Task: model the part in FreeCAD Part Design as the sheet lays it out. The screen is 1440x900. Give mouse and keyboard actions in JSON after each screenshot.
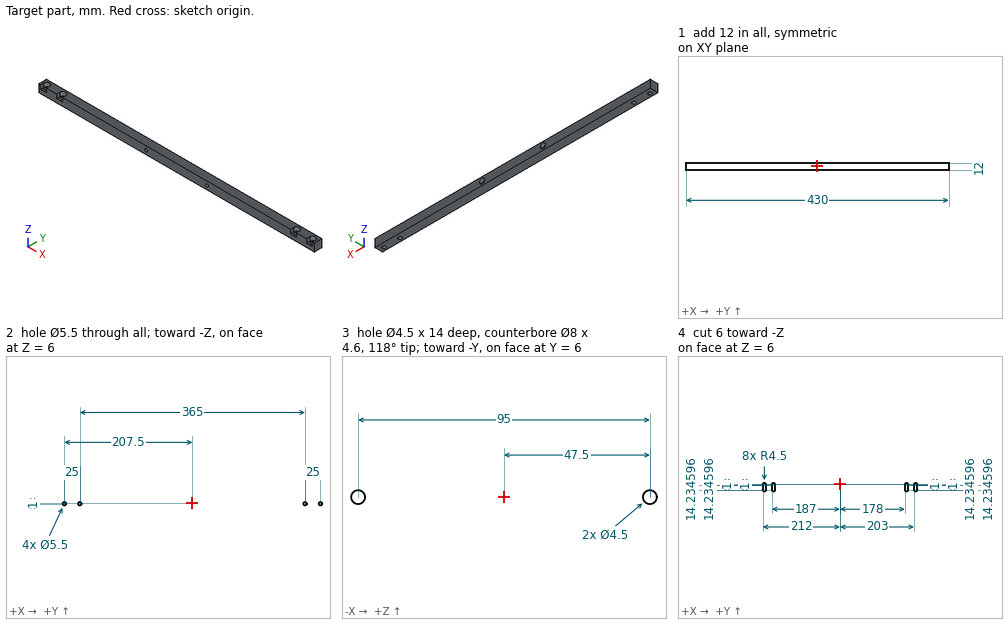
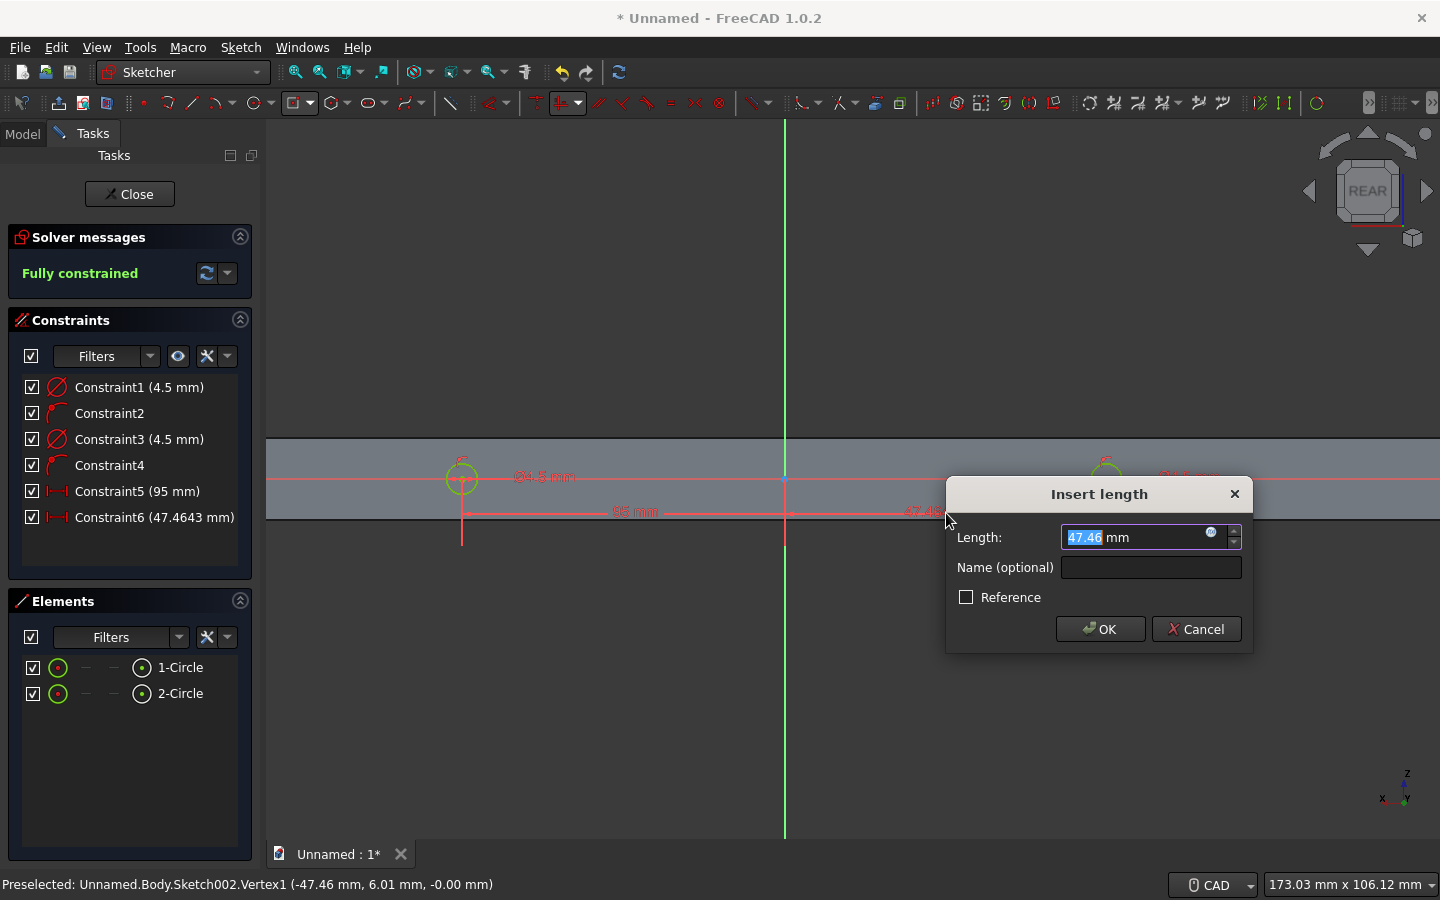
{"action": "type", "text": "47.5"}
{"action": "key", "text": "Return"}
{"action": "key", "text": "Escape"}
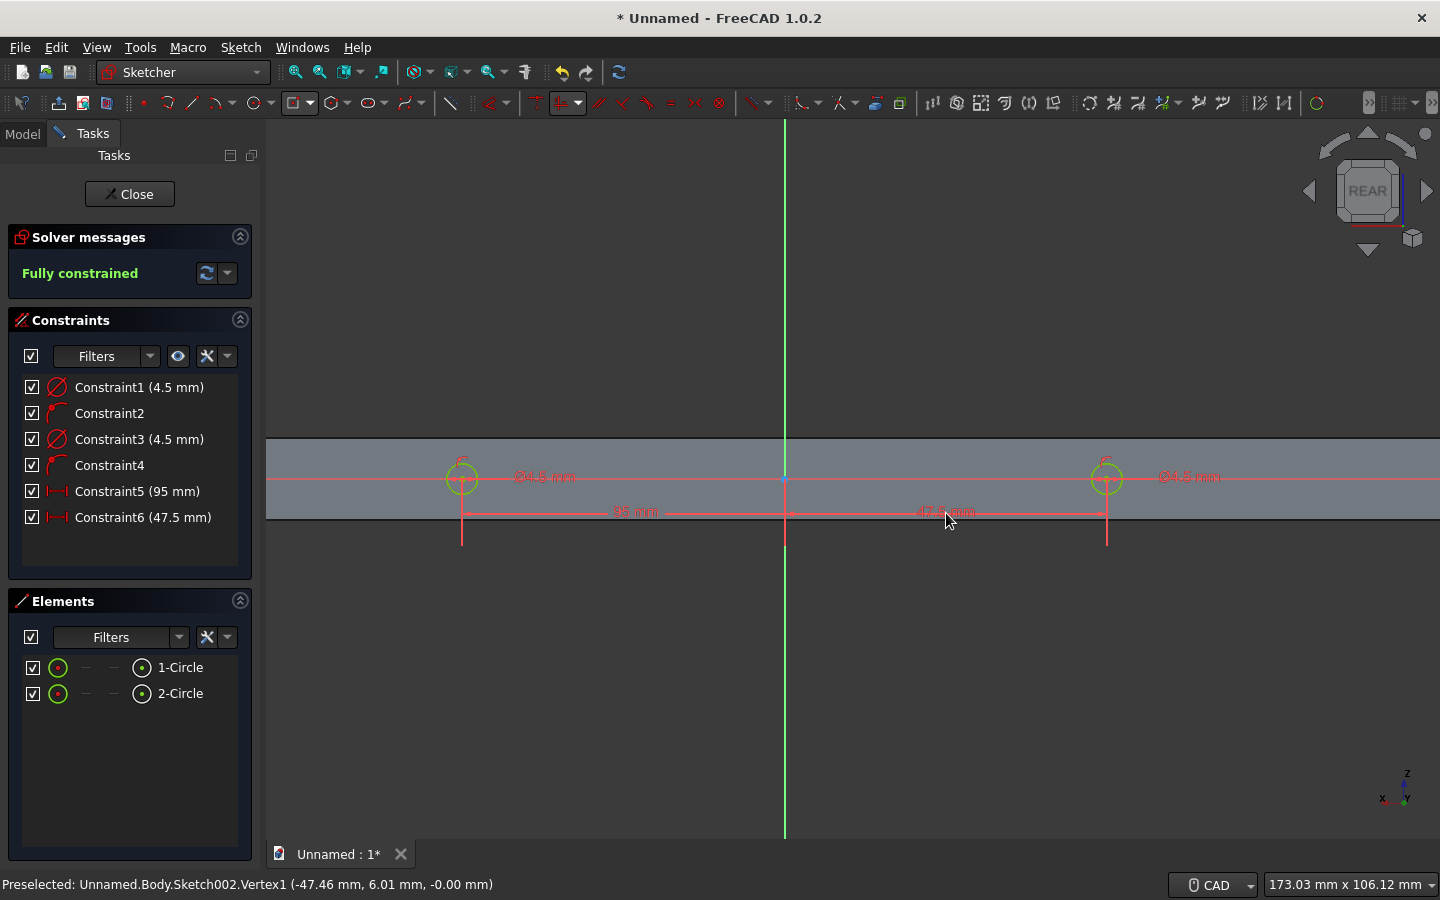
{"action": "left_click", "coordinate": [130, 194]}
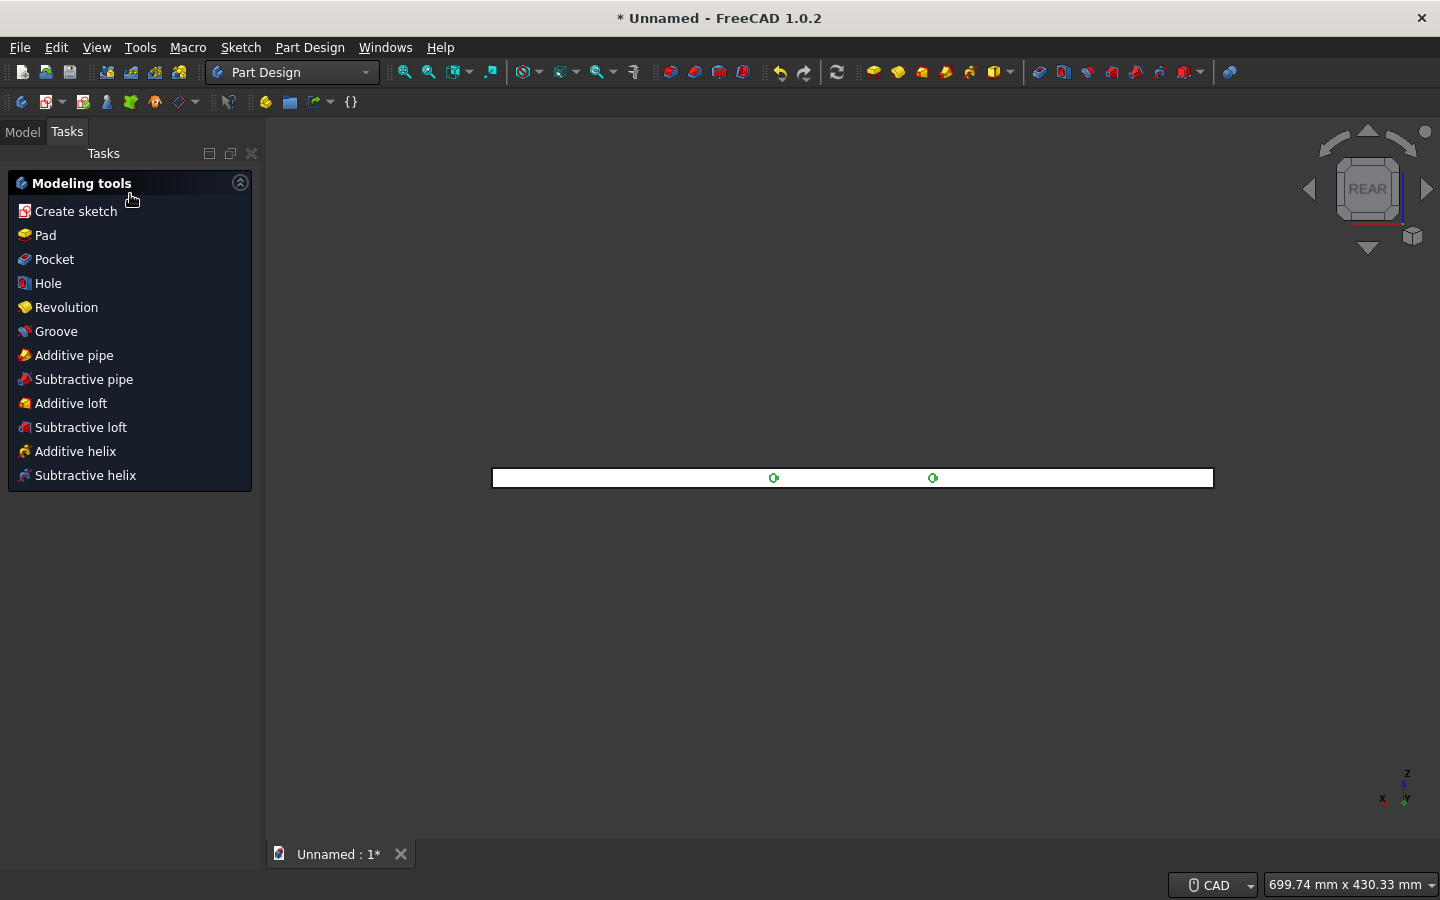
{"action": "left_click", "coordinate": [1064, 72]}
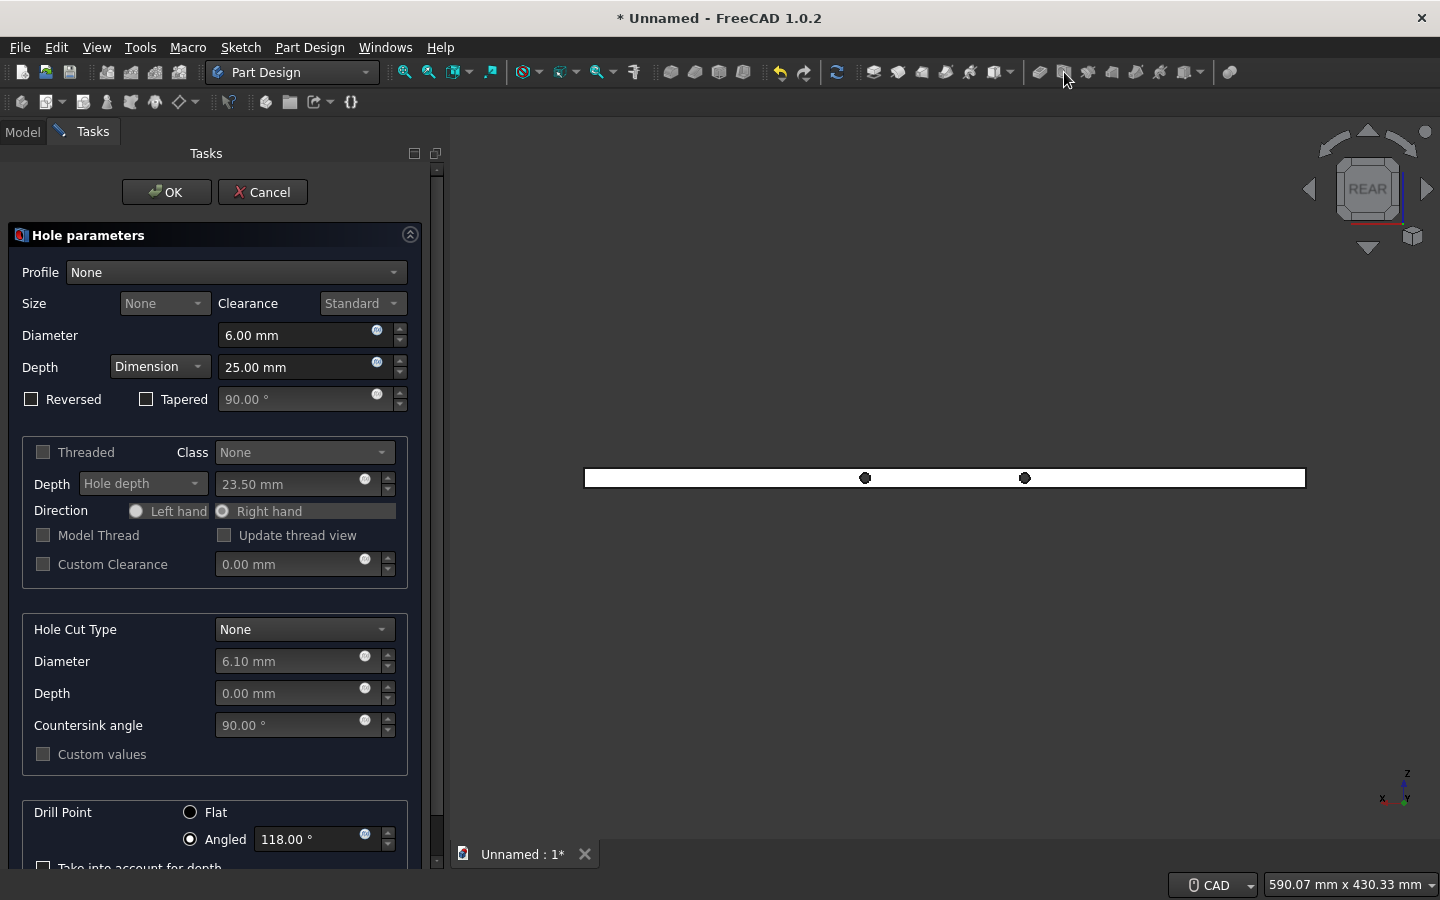
{"action": "triple_click", "coordinate": [305, 335]}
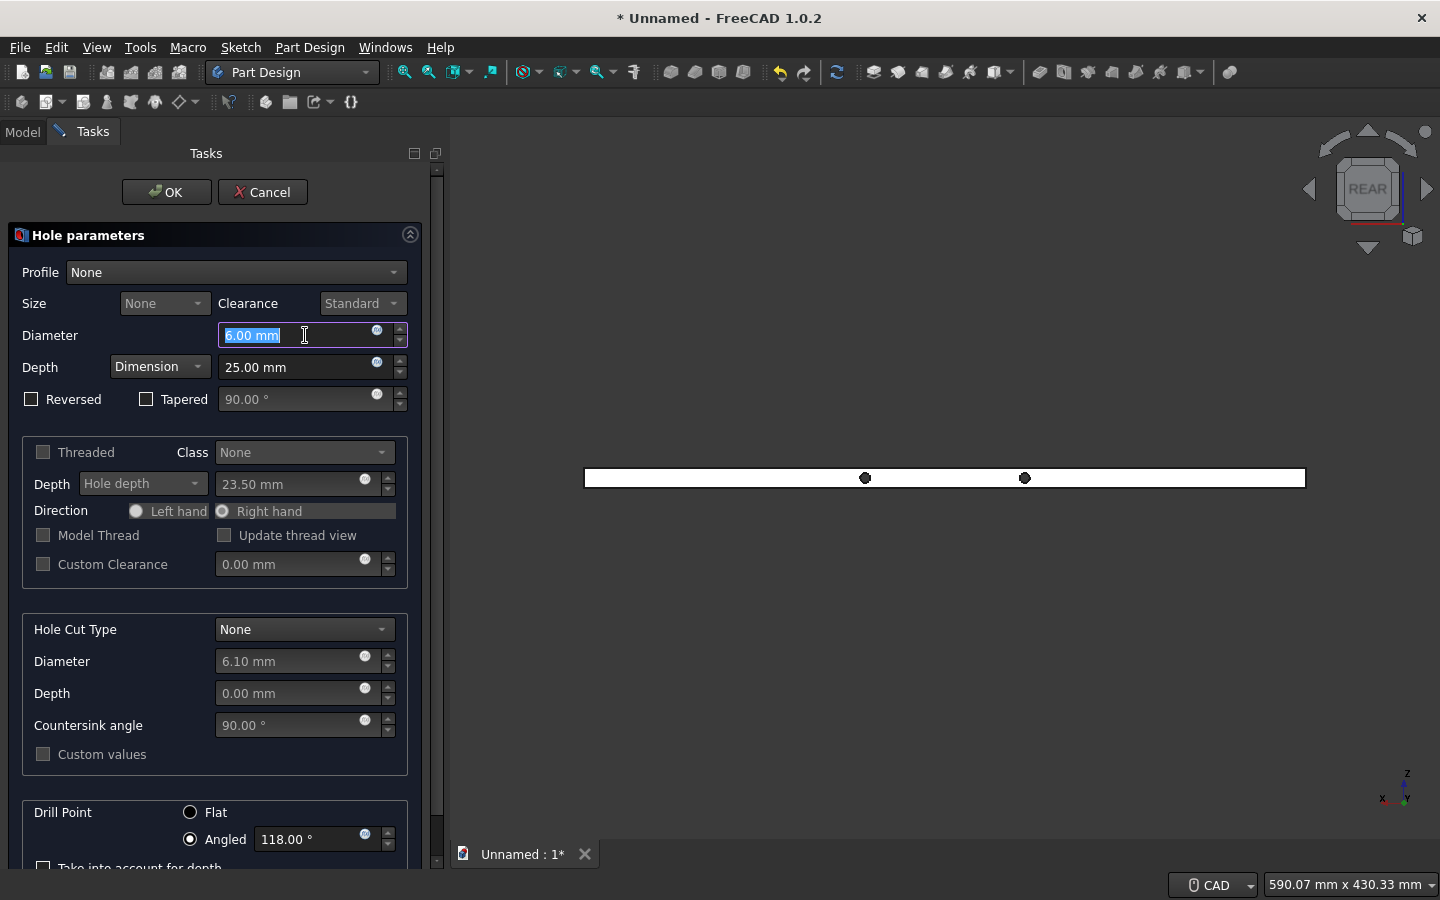
{"action": "type", "text": "4.5"}
{"action": "key", "text": "Tab"}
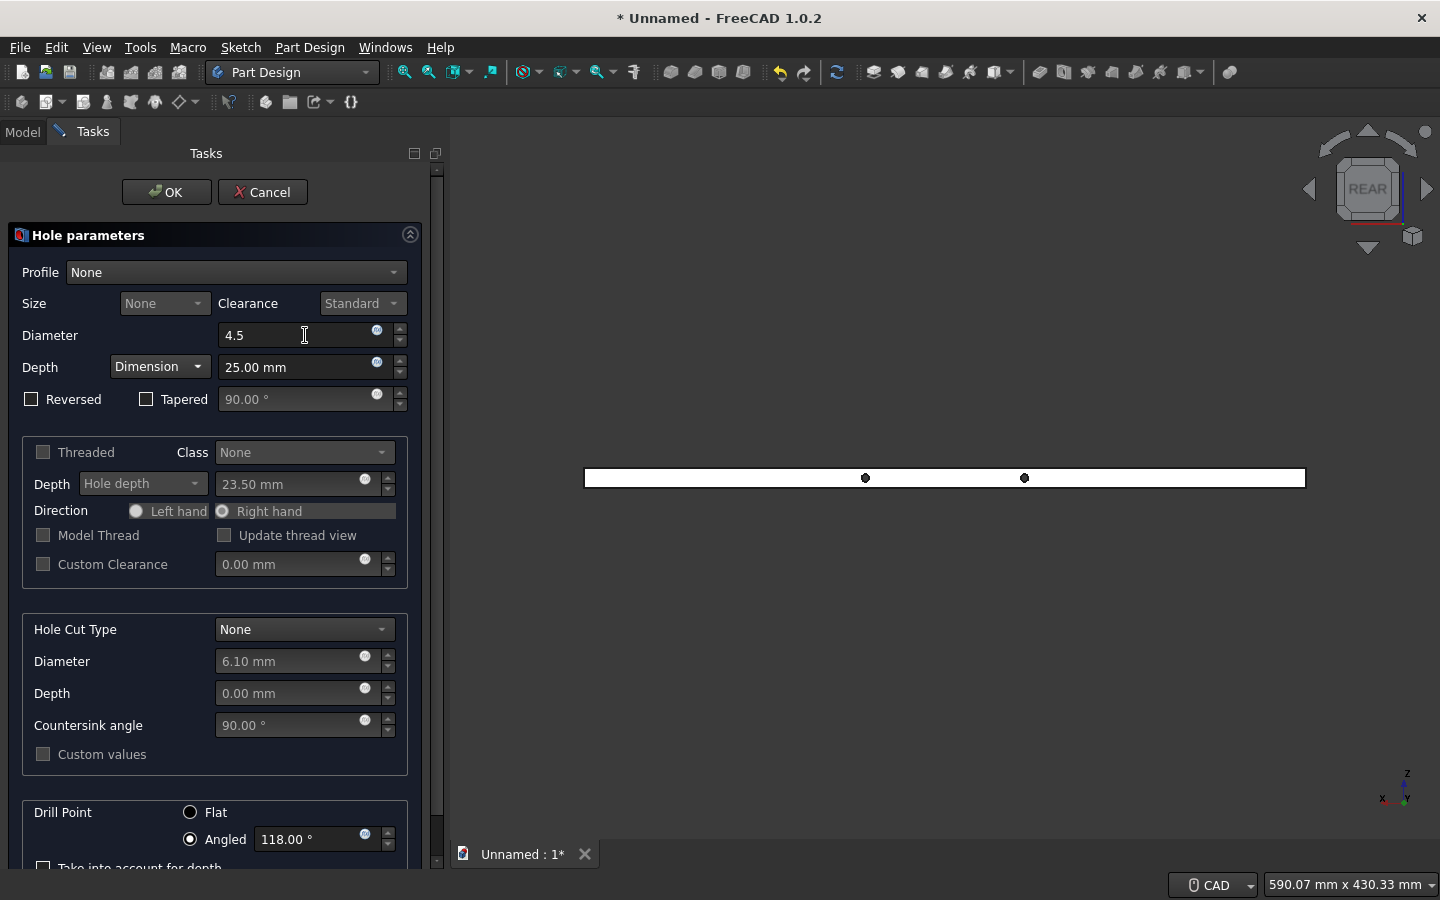
{"action": "triple_click", "coordinate": [305, 367]}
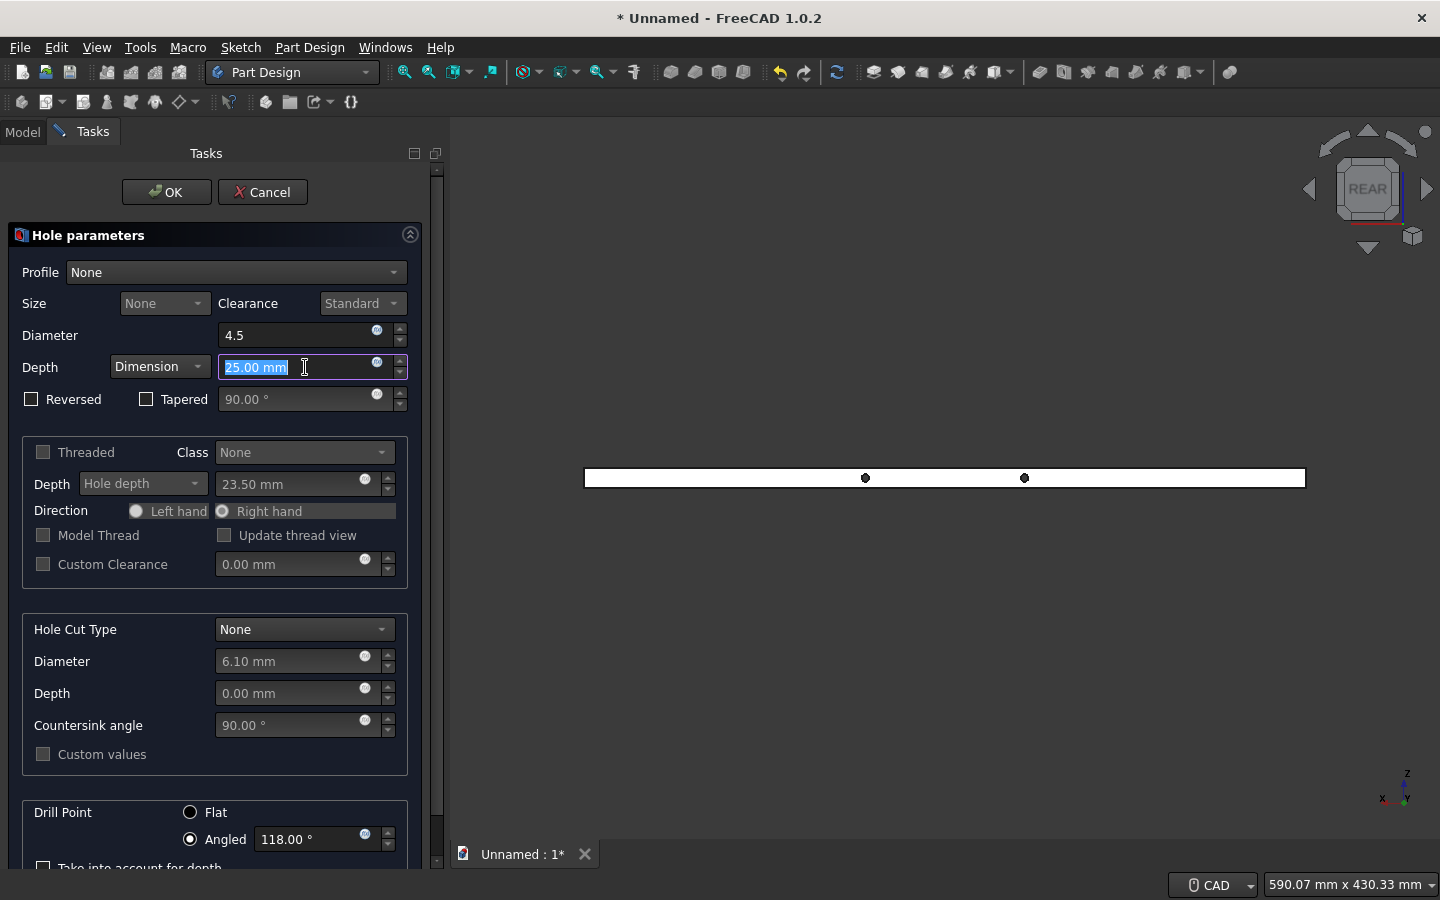
{"action": "type", "text": "14"}
{"action": "key", "text": "Tab"}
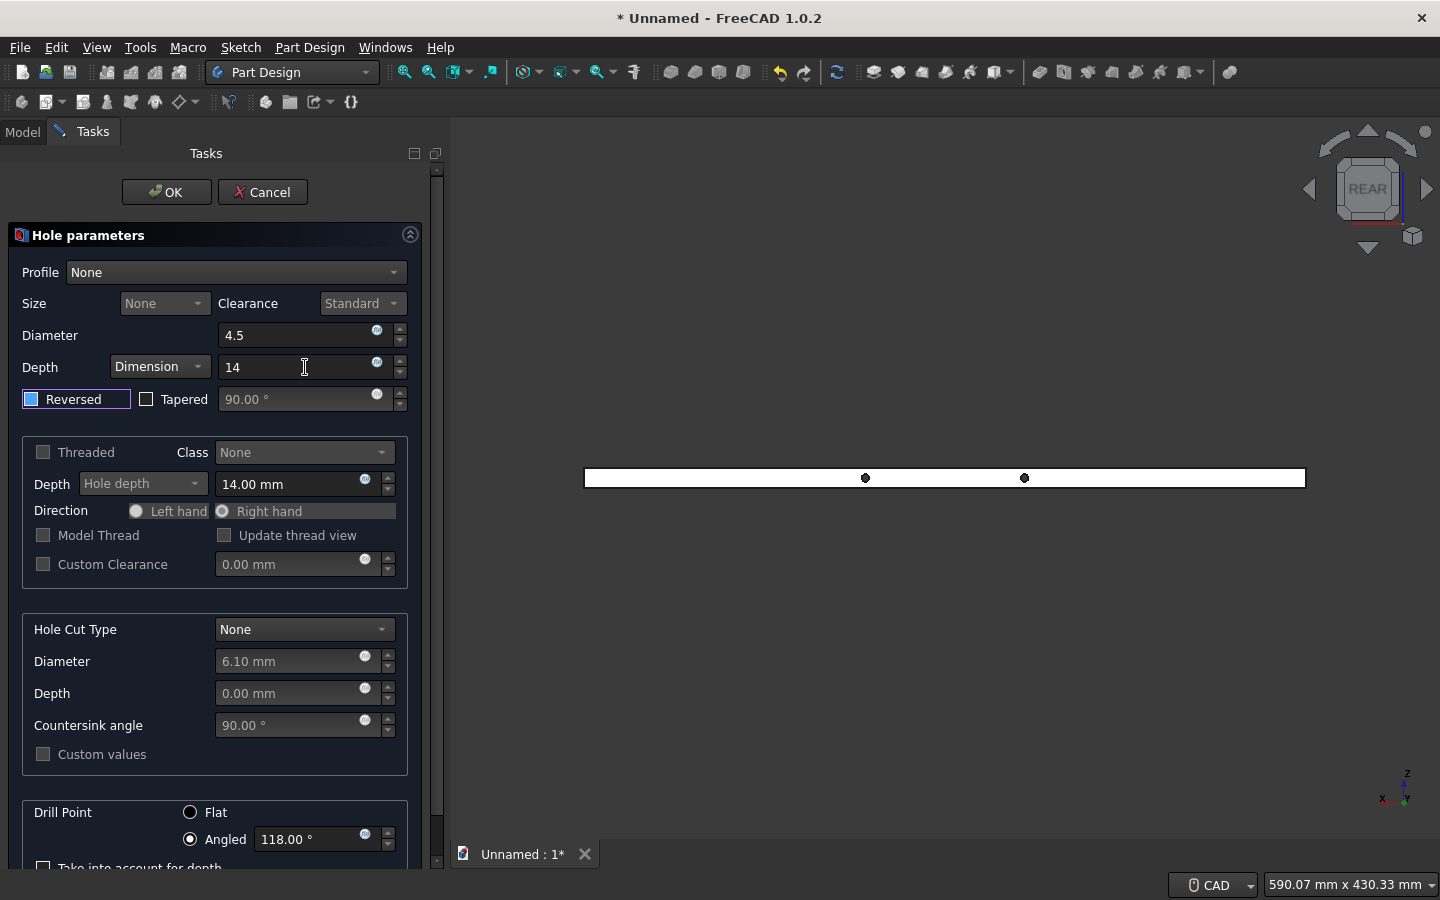
{"action": "left_click", "coordinate": [306, 630]}